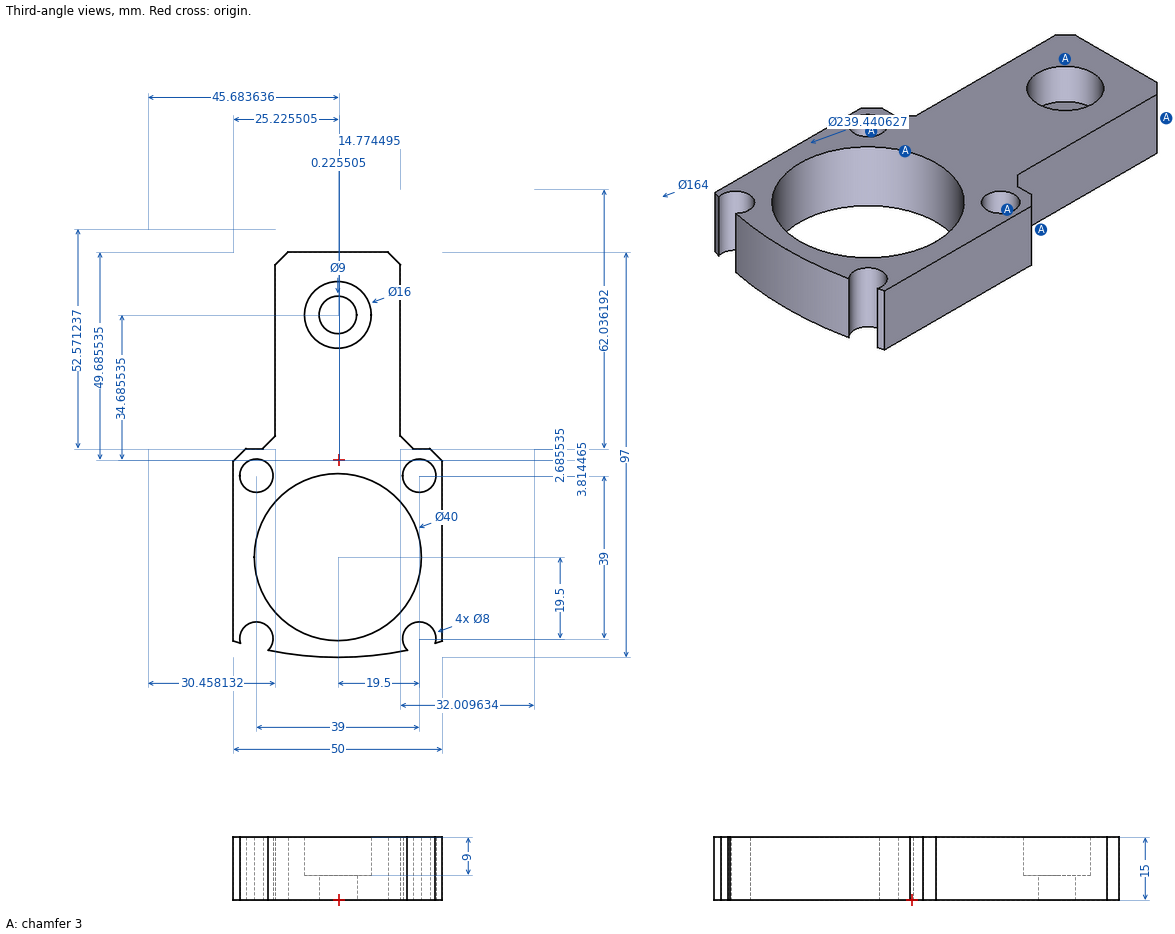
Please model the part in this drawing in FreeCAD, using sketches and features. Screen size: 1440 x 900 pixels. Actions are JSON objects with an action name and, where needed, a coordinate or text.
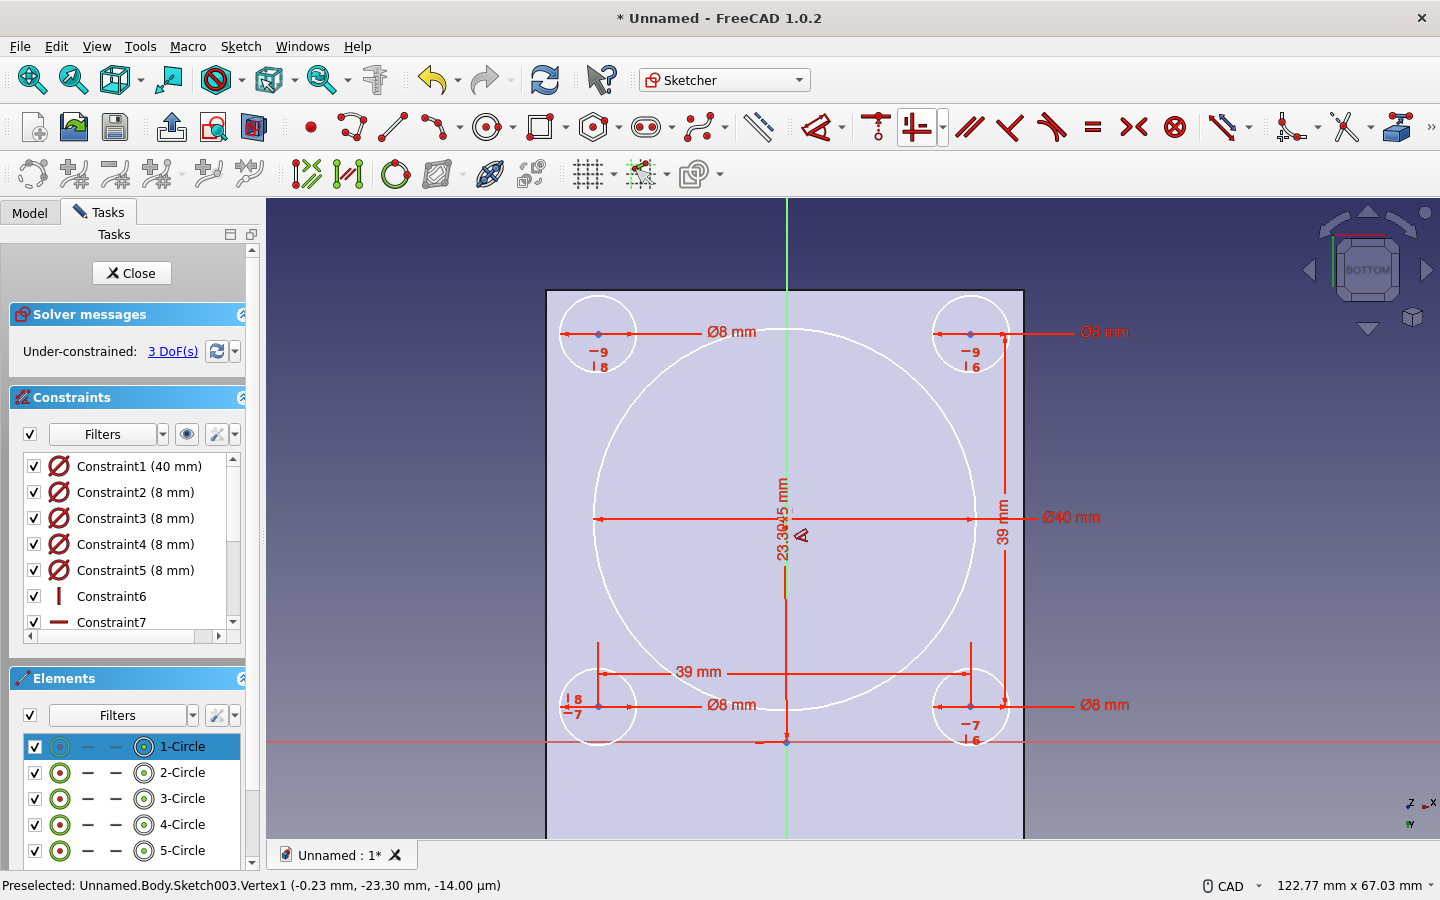
{"action": "left_click", "coordinate": [971, 334]}
{"action": "left_click", "coordinate": [878, 300]}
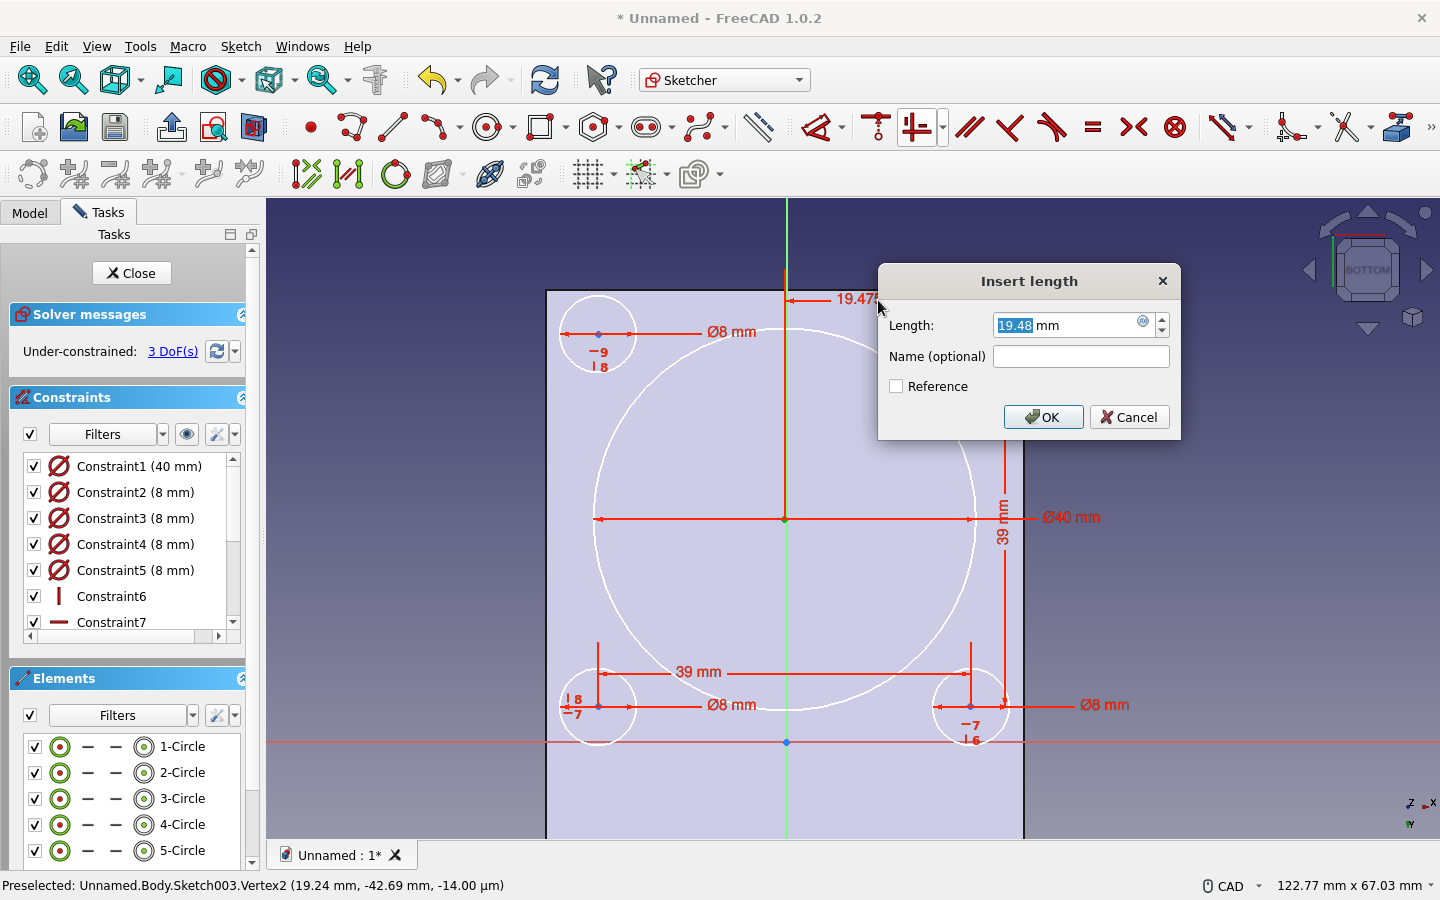
{"action": "type", "text": "19.5"}
{"action": "key", "text": "Return"}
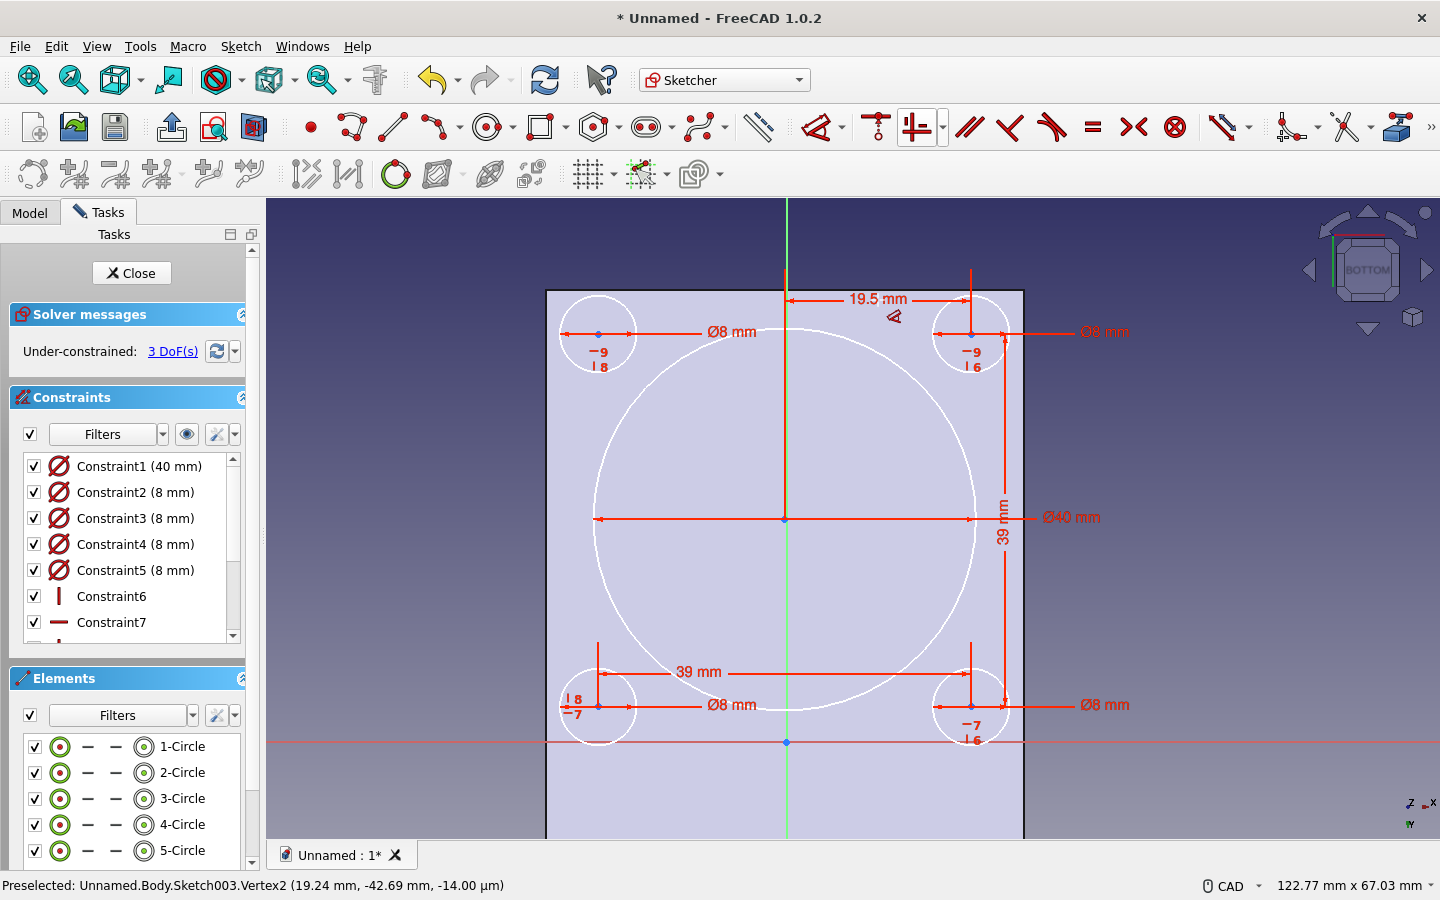
{"action": "left_click", "coordinate": [785, 519]}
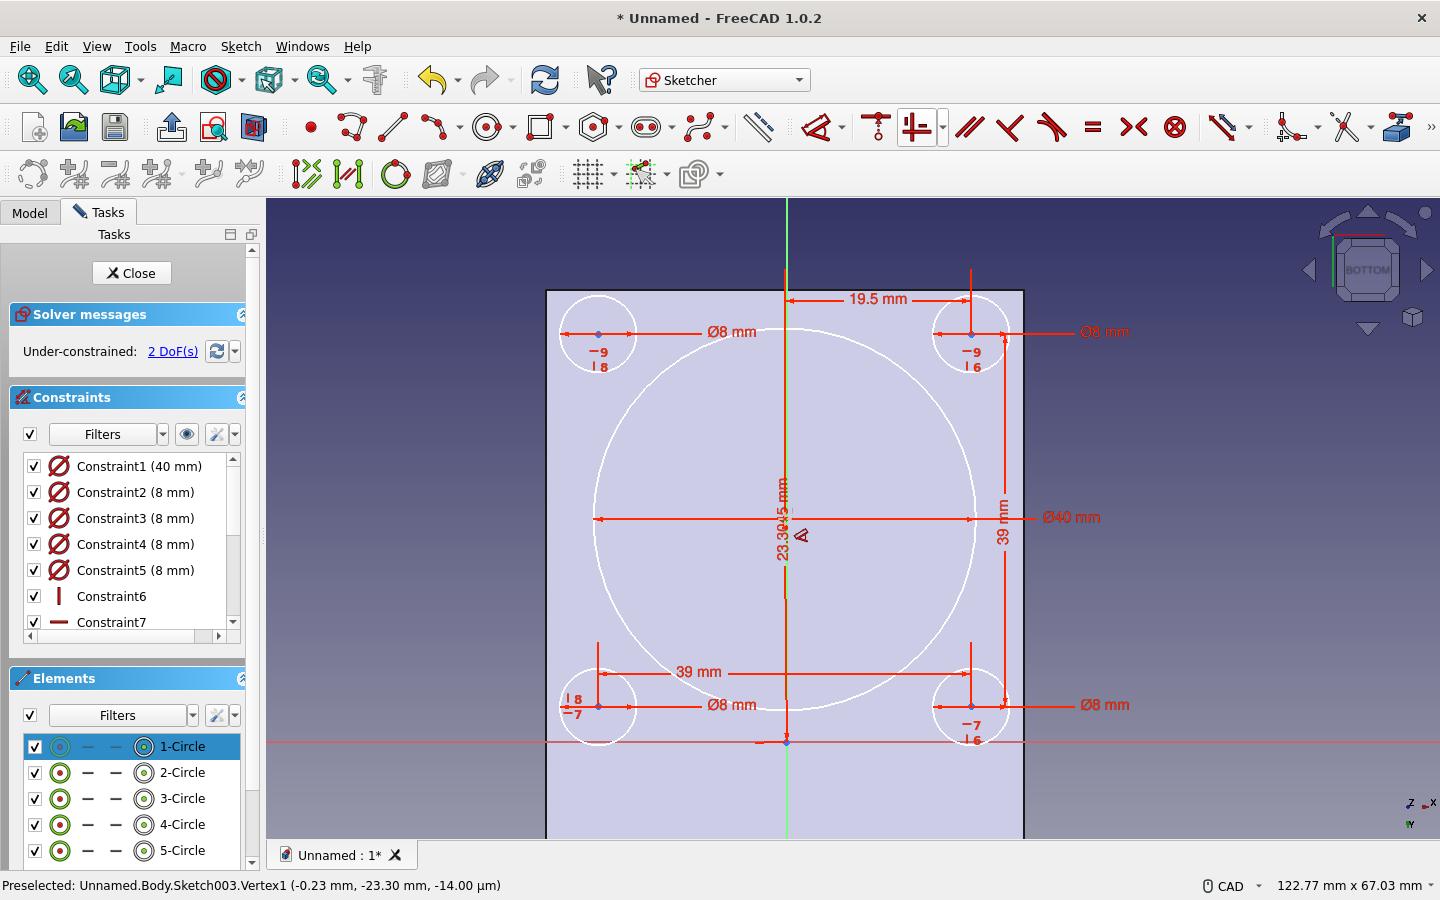
{"action": "left_click", "coordinate": [971, 334]}
{"action": "left_click", "coordinate": [1005, 427]}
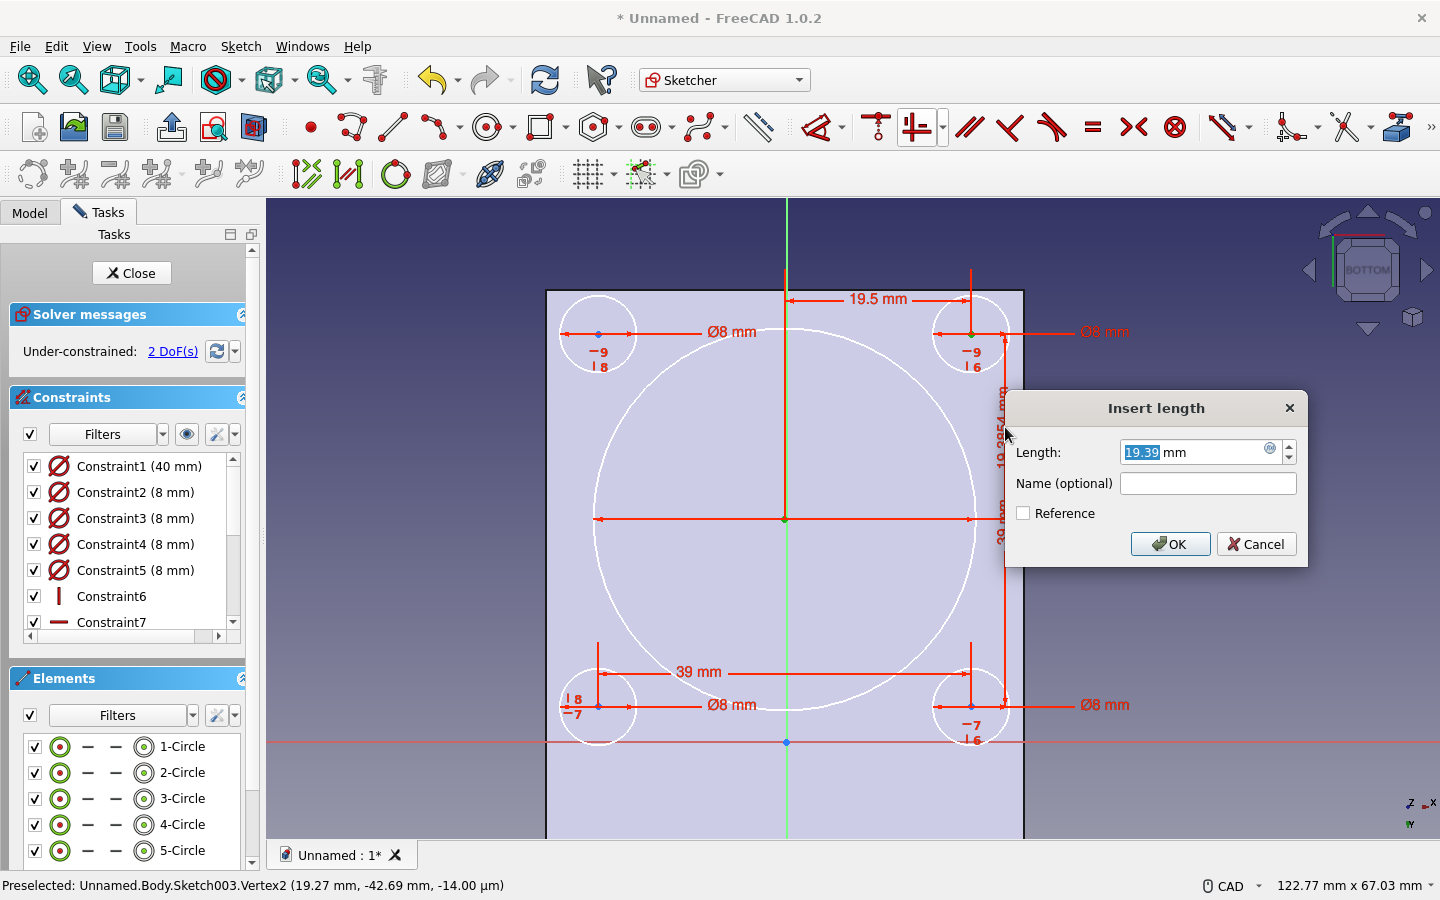
{"action": "type", "text": "19.5"}
{"action": "key", "text": "Return"}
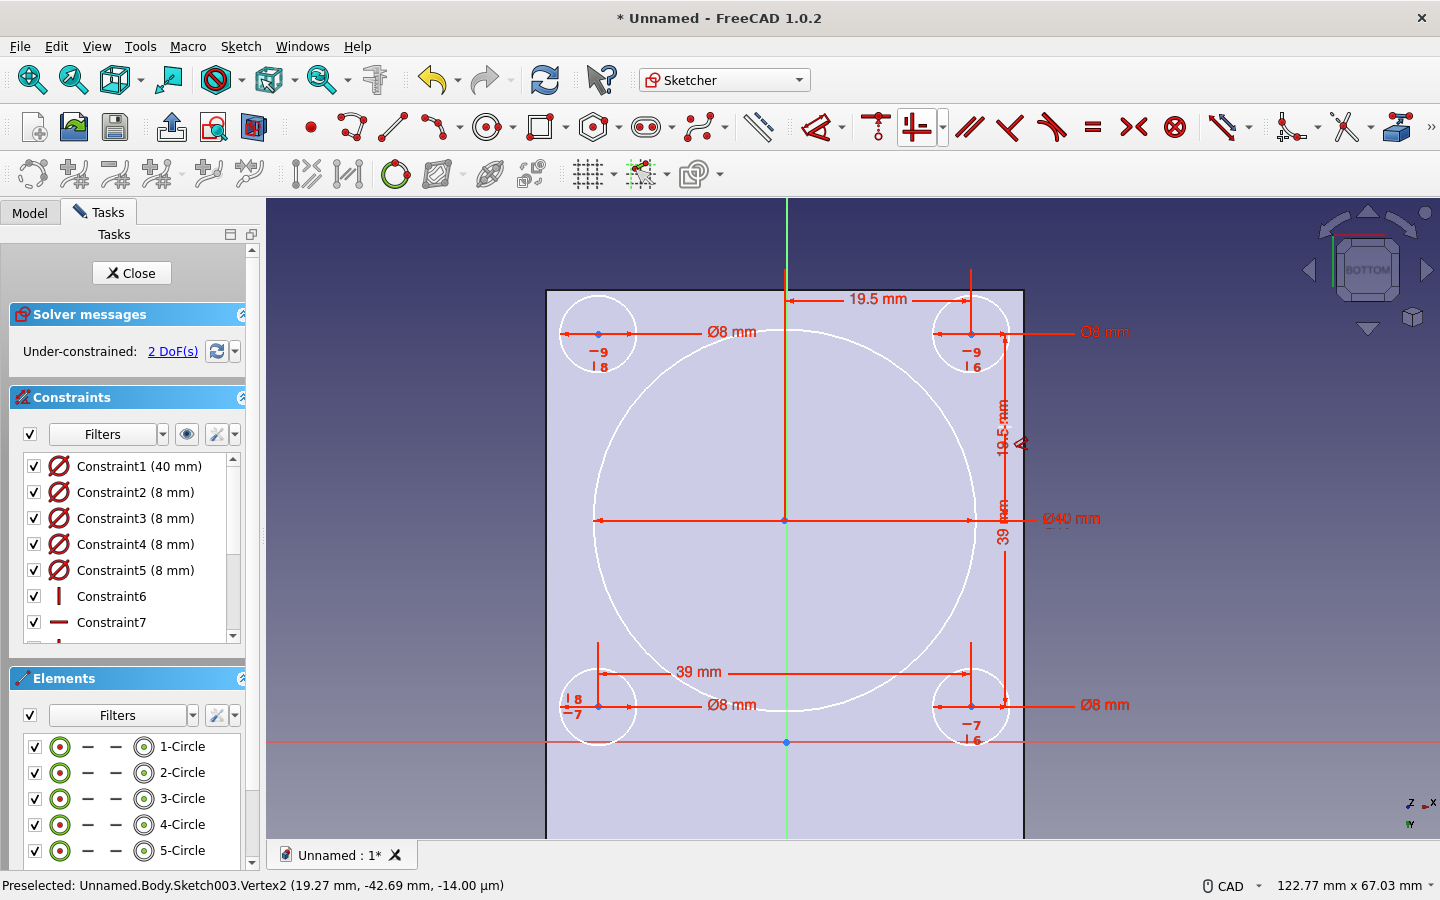
{"action": "scroll", "coordinate": [785, 521], "scroll_direction": "up", "scroll_amount": 15}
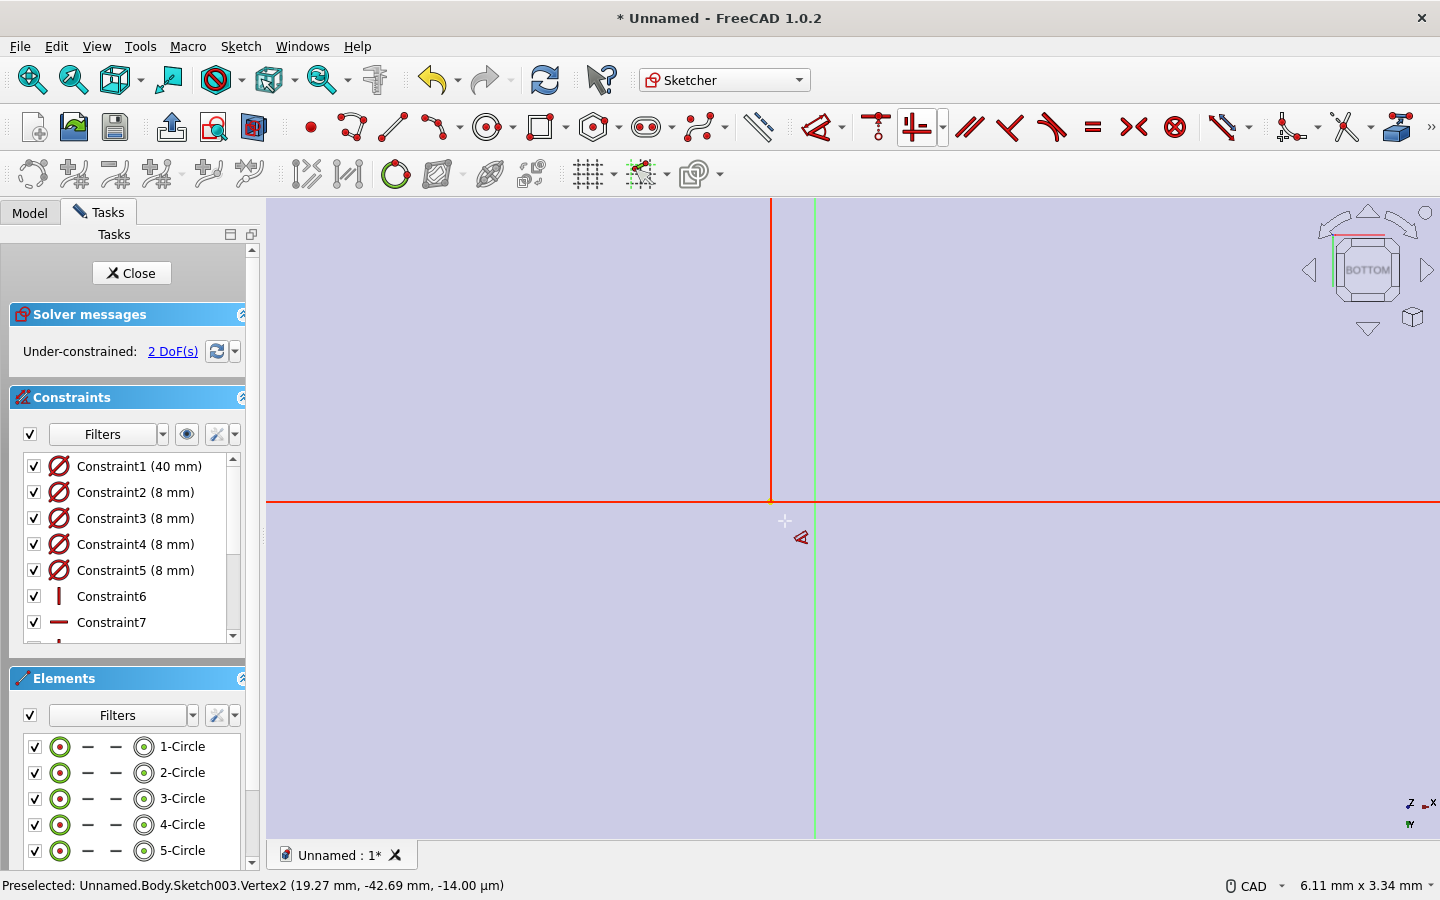
{"action": "left_click", "coordinate": [771, 502]}
{"action": "left_click", "coordinate": [793, 468]}